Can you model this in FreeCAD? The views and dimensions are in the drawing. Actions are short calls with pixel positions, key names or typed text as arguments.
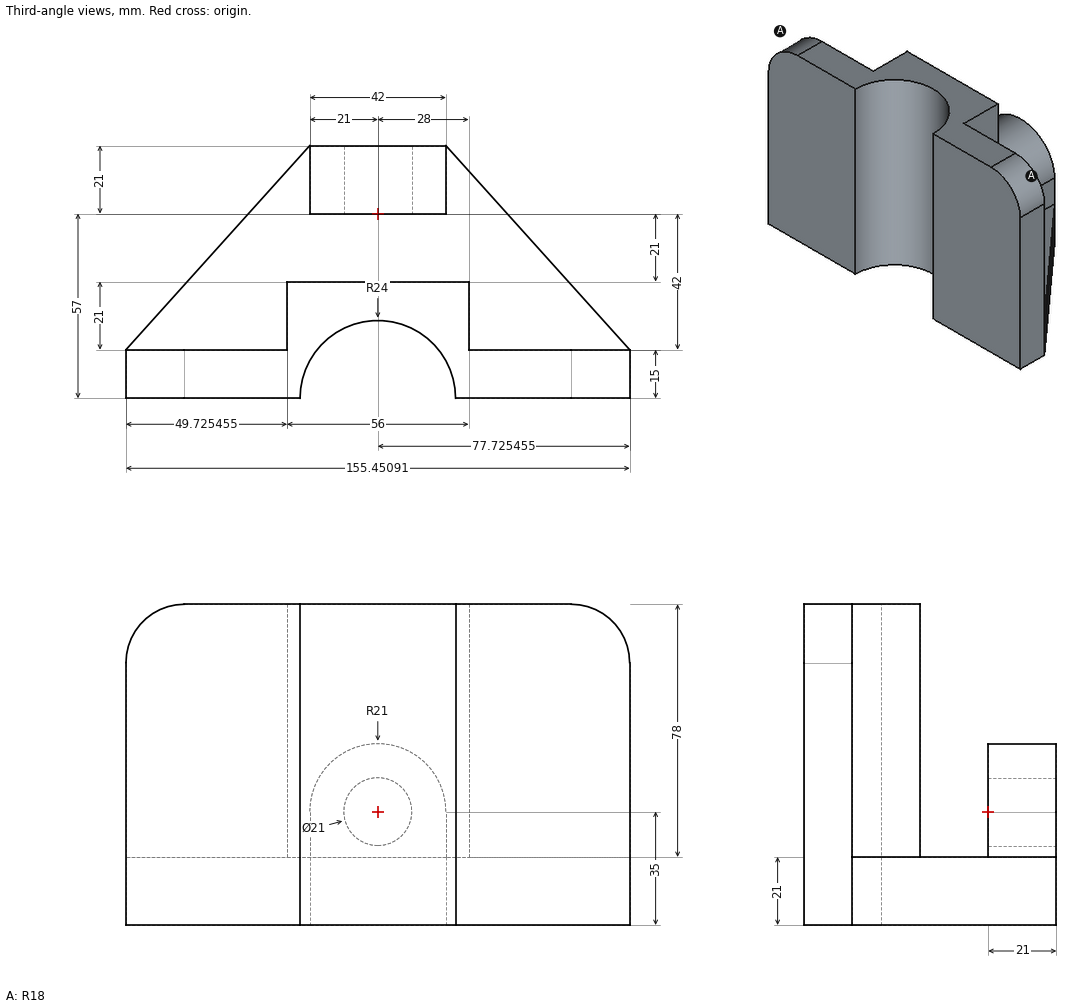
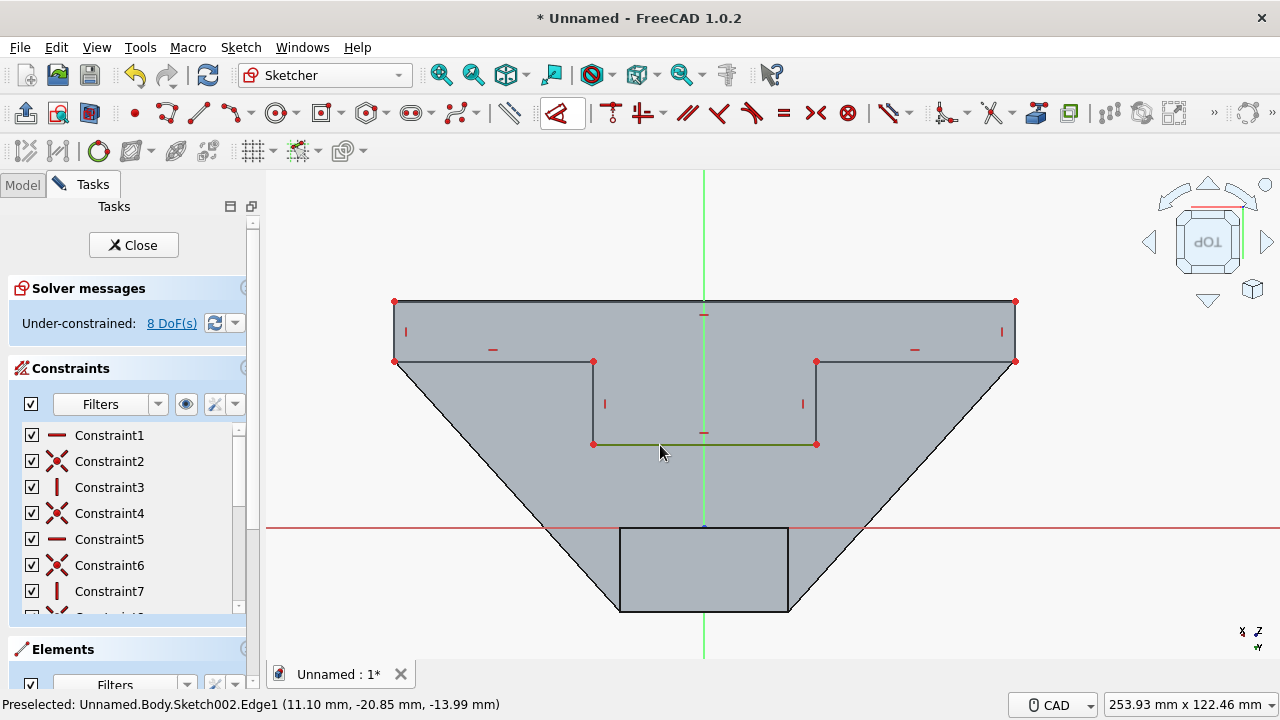
click(580, 114)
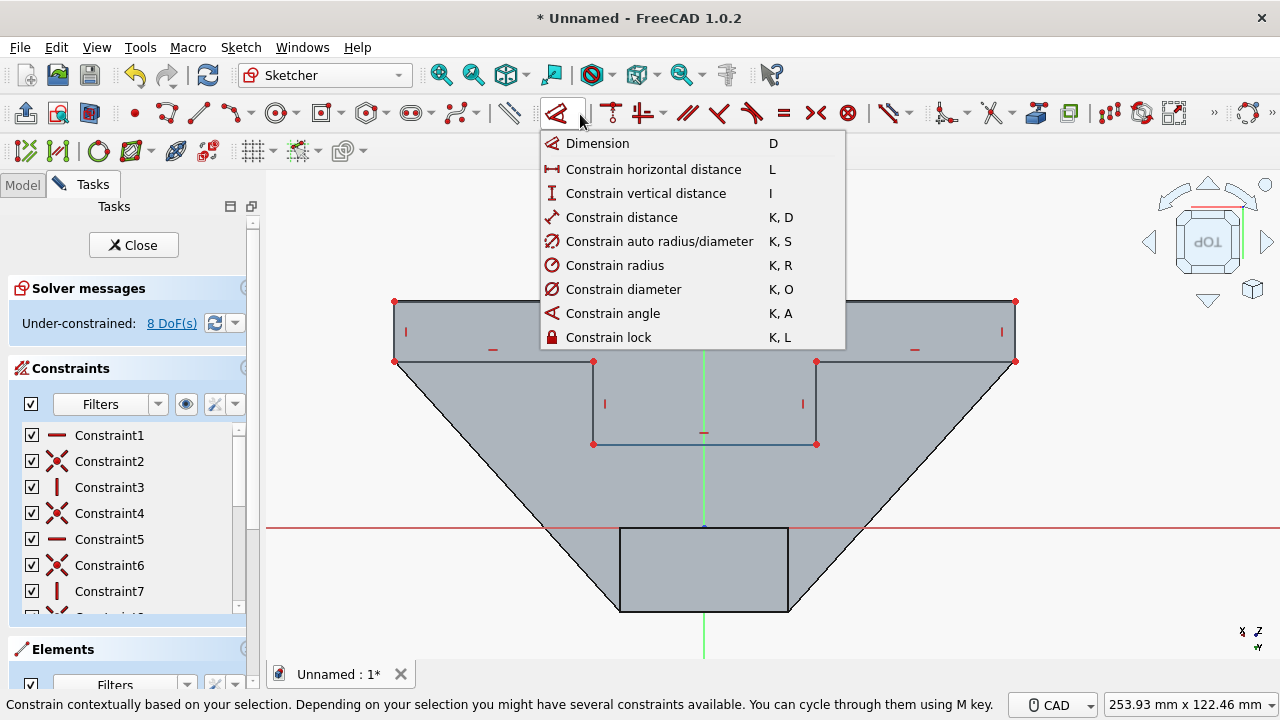
click(693, 169)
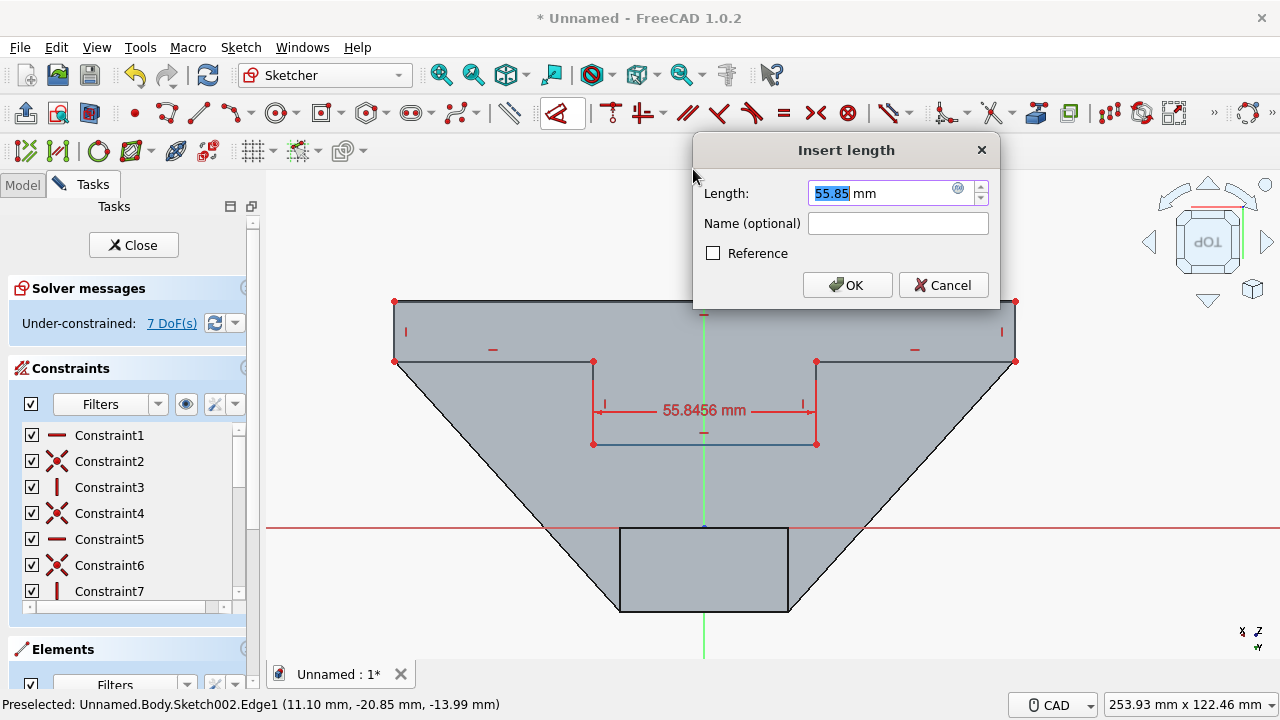
text(56)
key(Return)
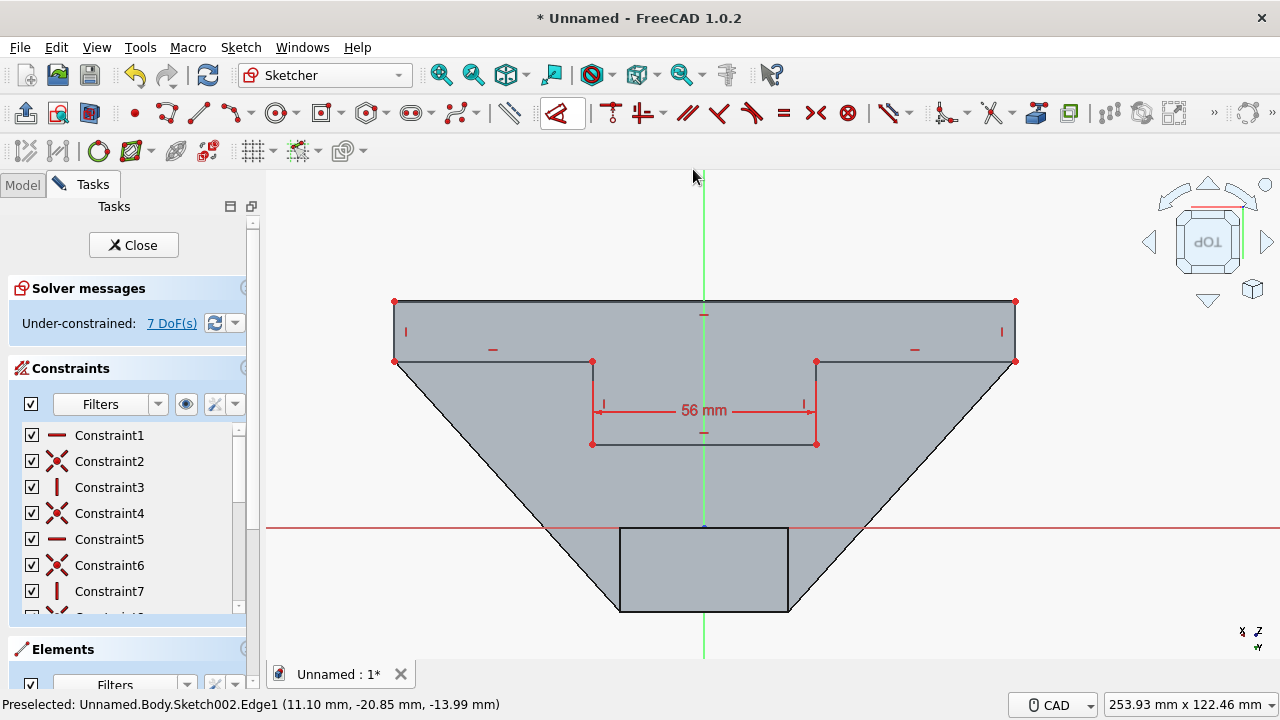
click(816, 420)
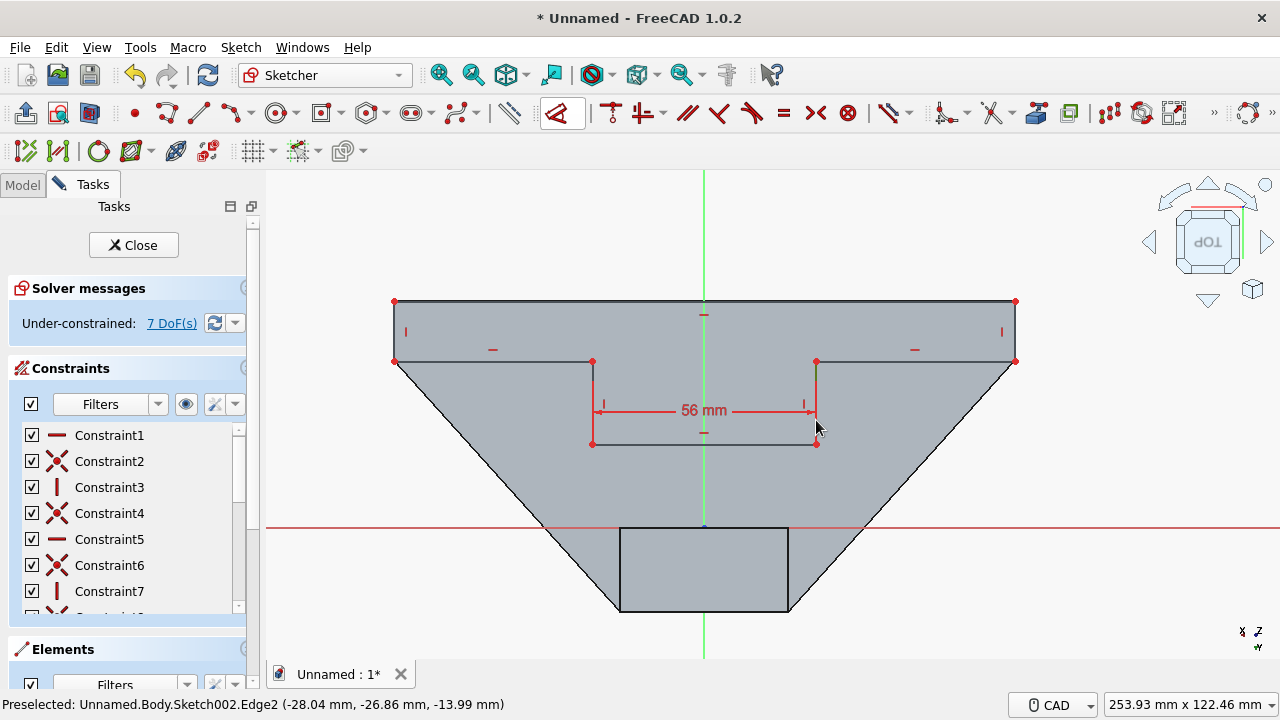
click(580, 114)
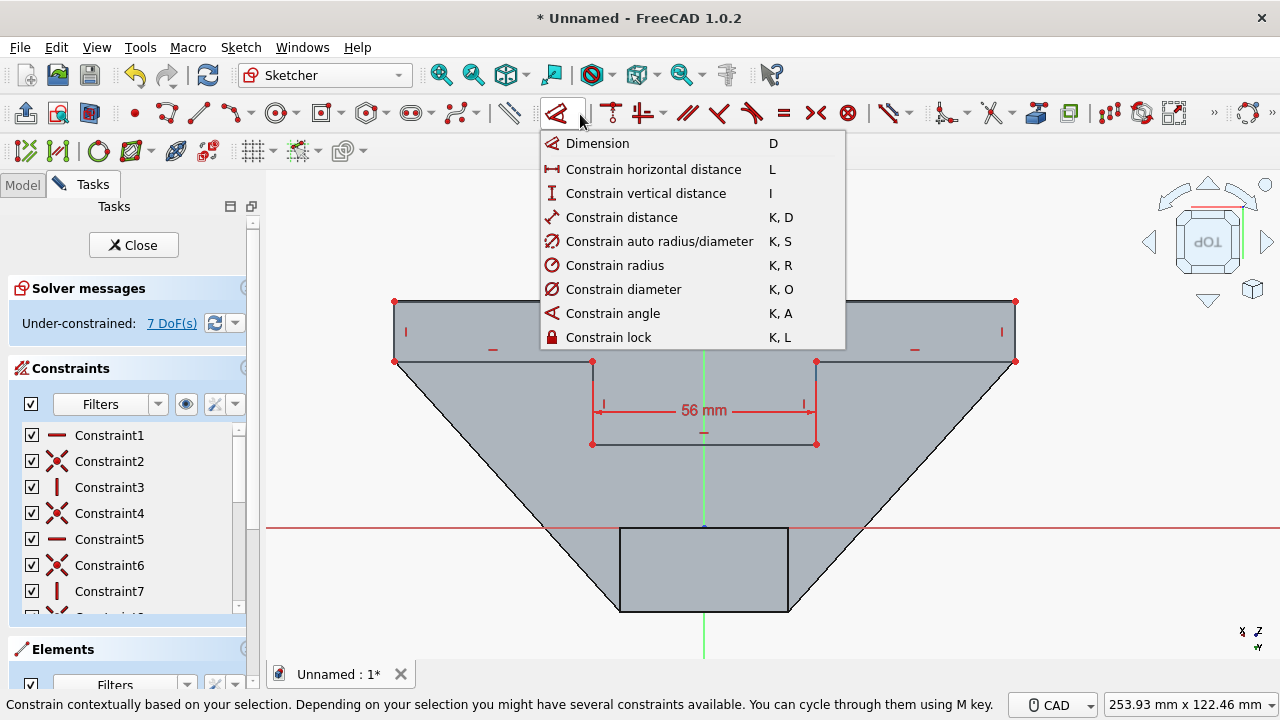
click(693, 193)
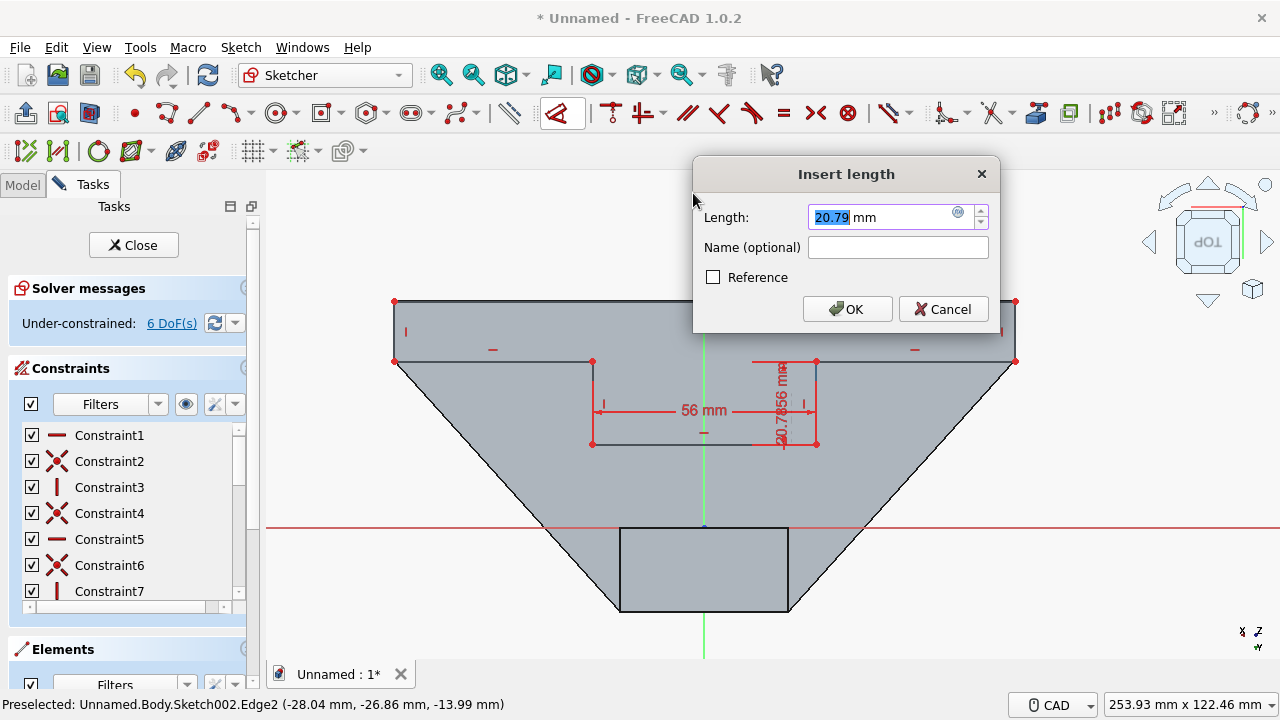
text(21)
key(Return)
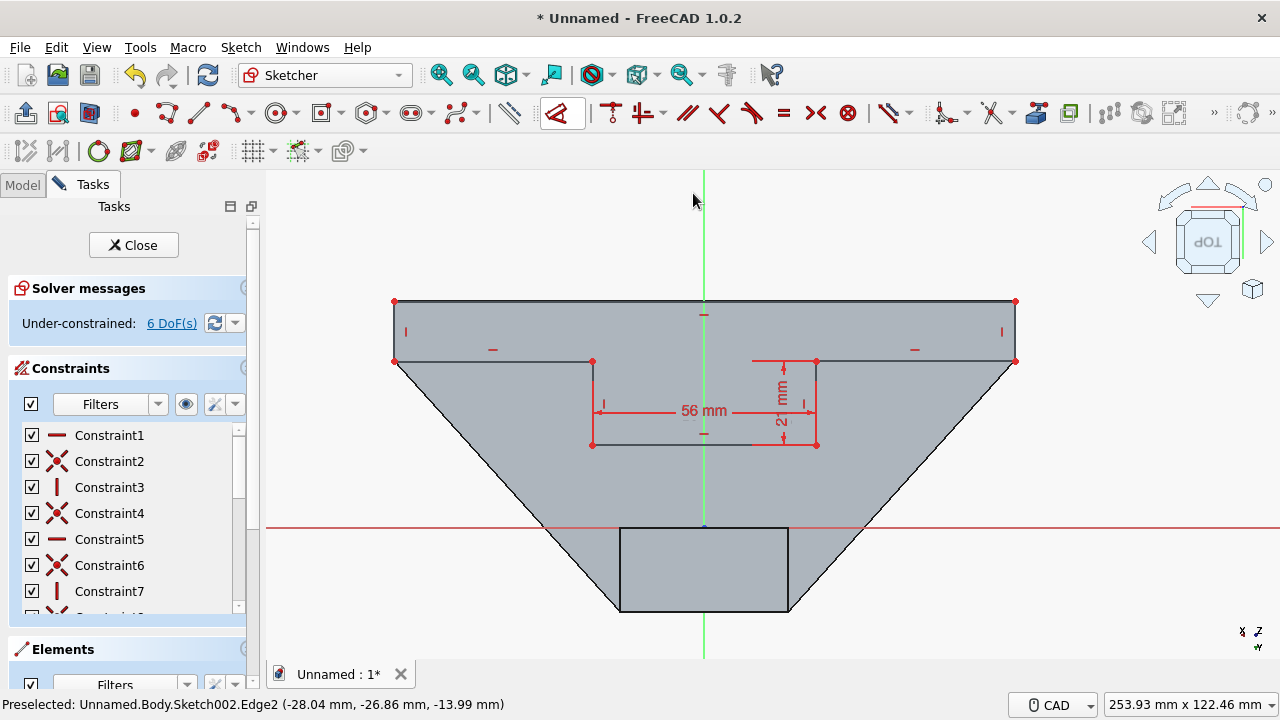
click(1015, 344)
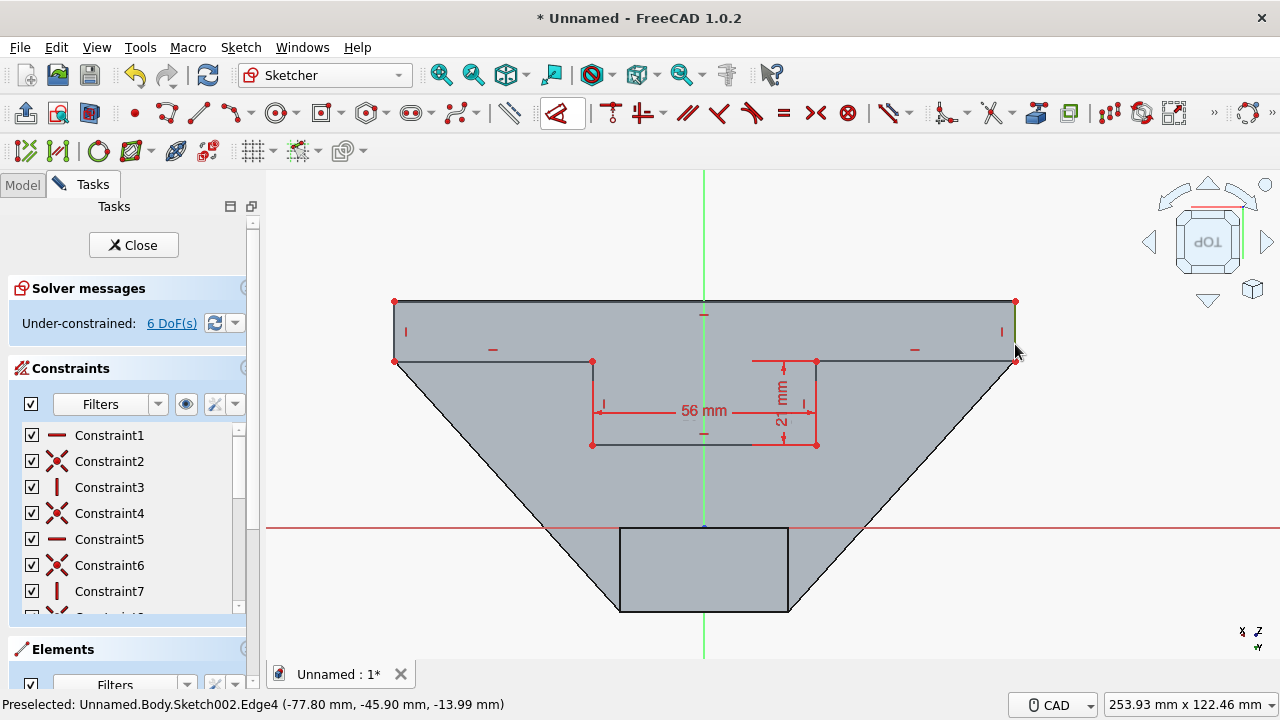
key(i)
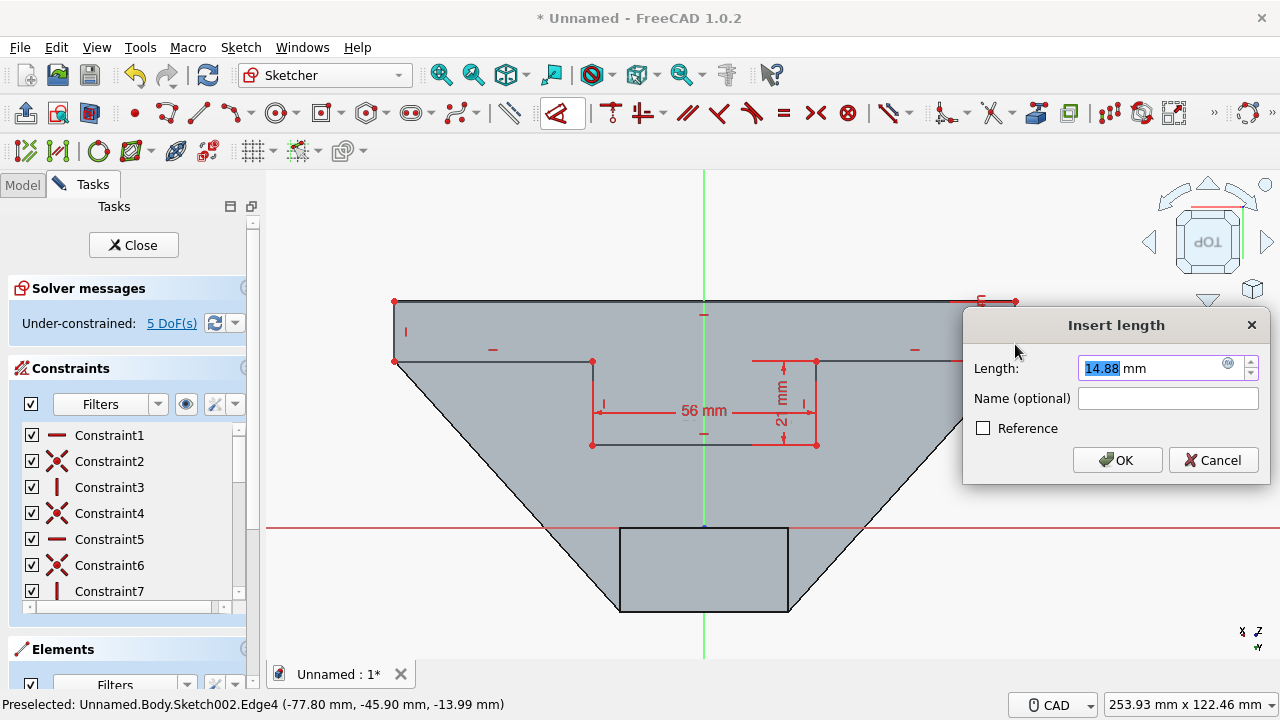
text(15)
key(Return)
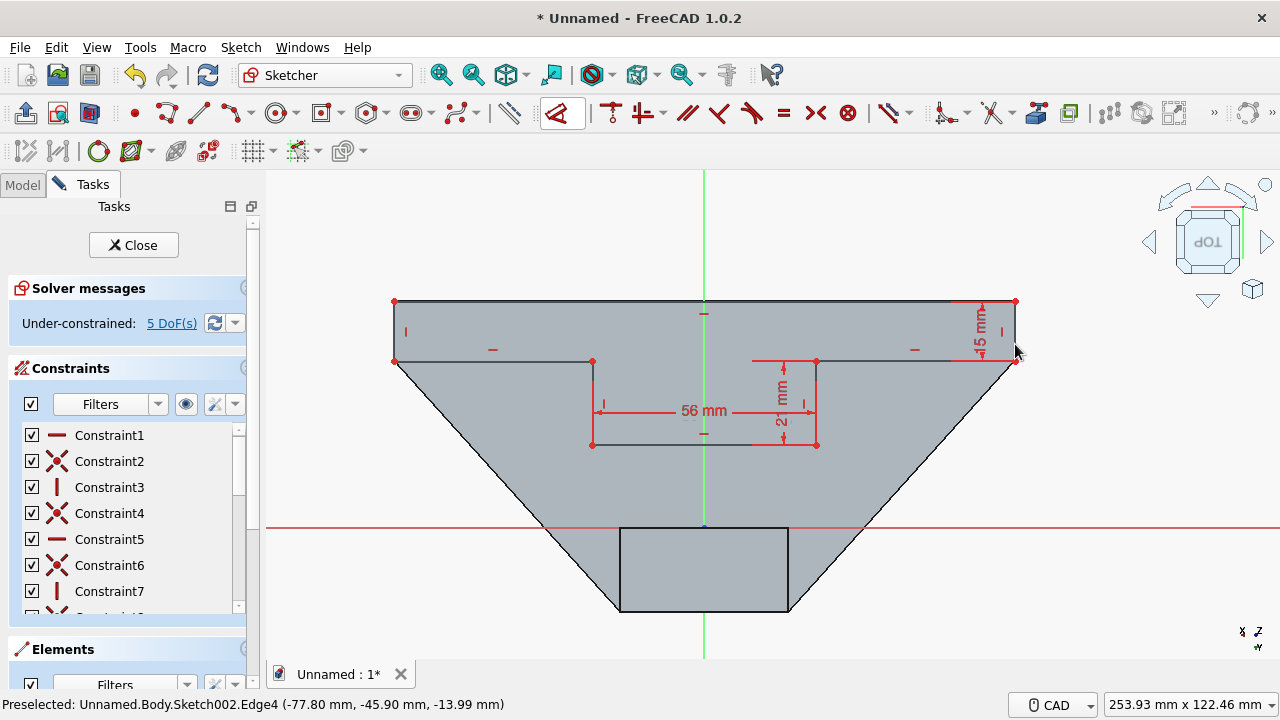
click(394, 320)